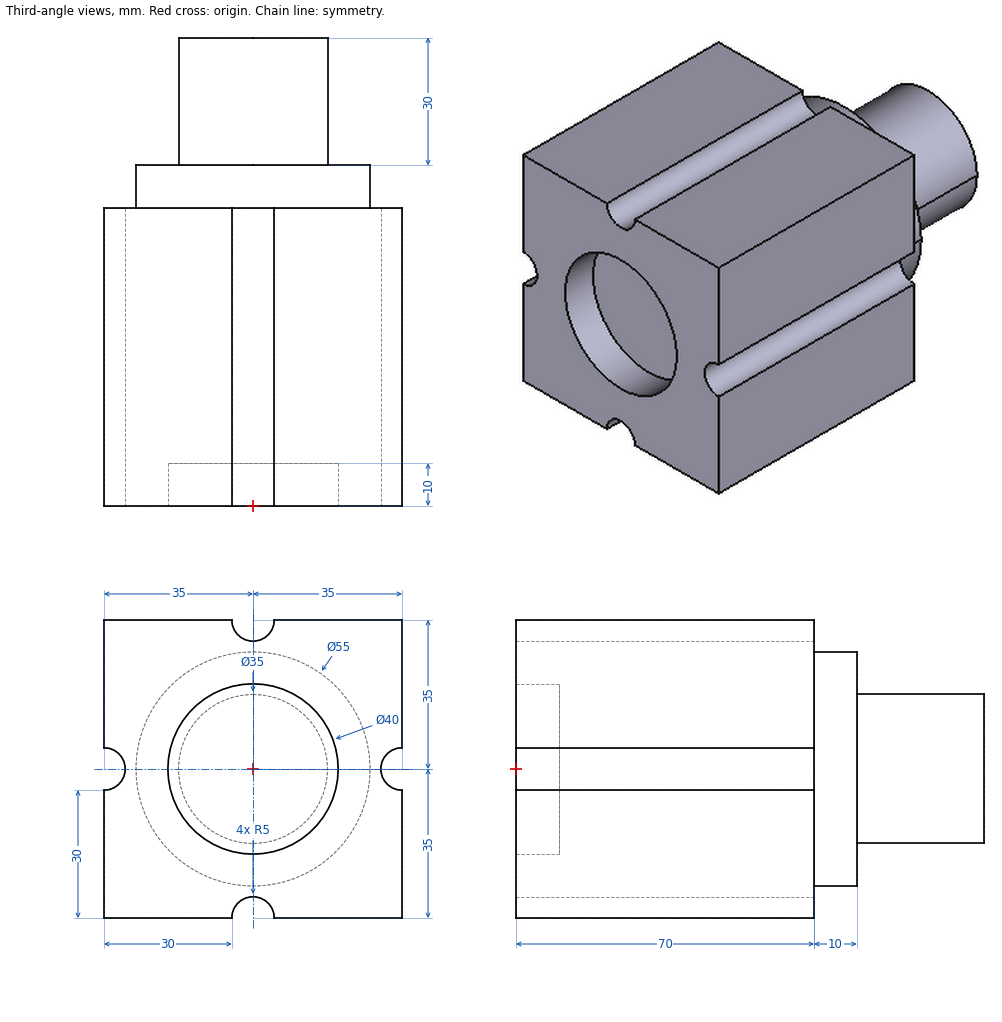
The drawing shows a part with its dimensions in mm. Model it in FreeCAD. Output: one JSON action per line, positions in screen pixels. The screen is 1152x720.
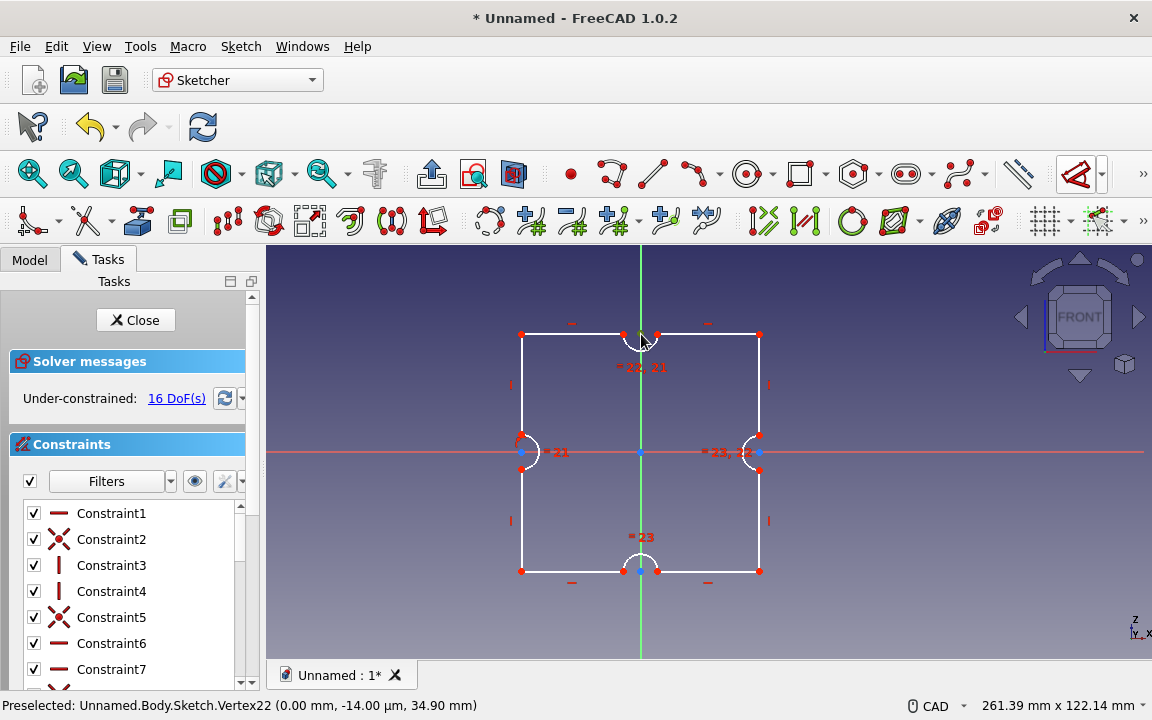
{"action": "left_click", "coordinate": [641, 605]}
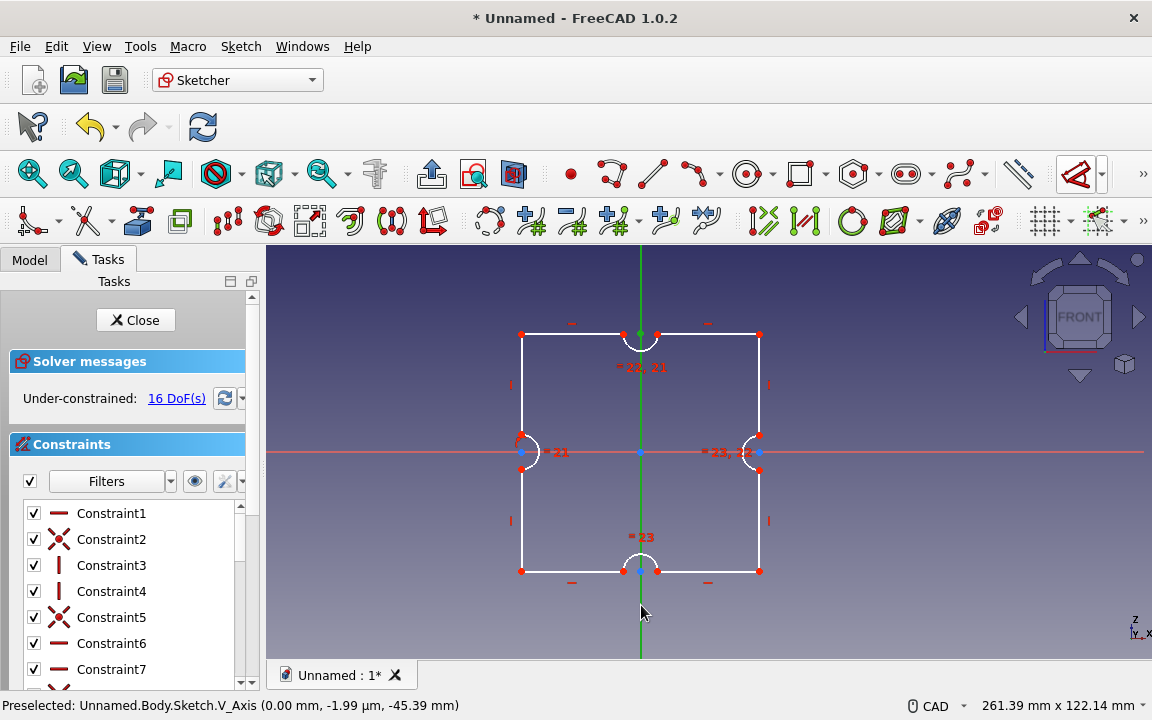
{"action": "key", "text": "c"}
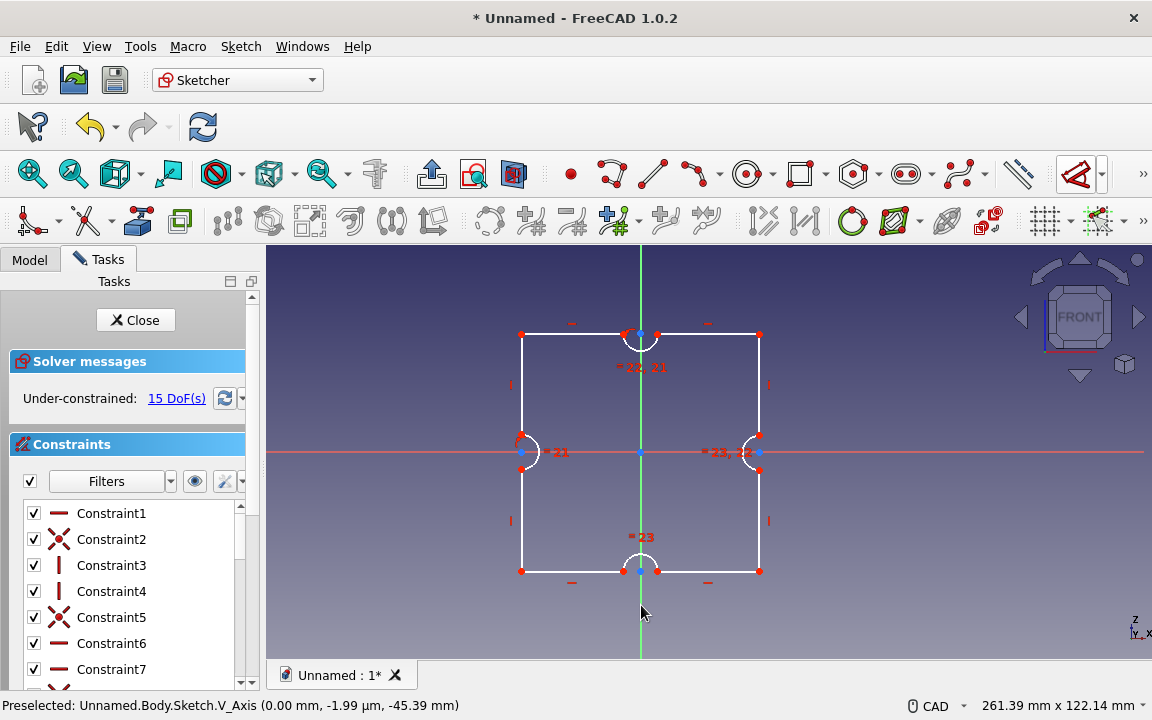
{"action": "left_click", "coordinate": [760, 453]}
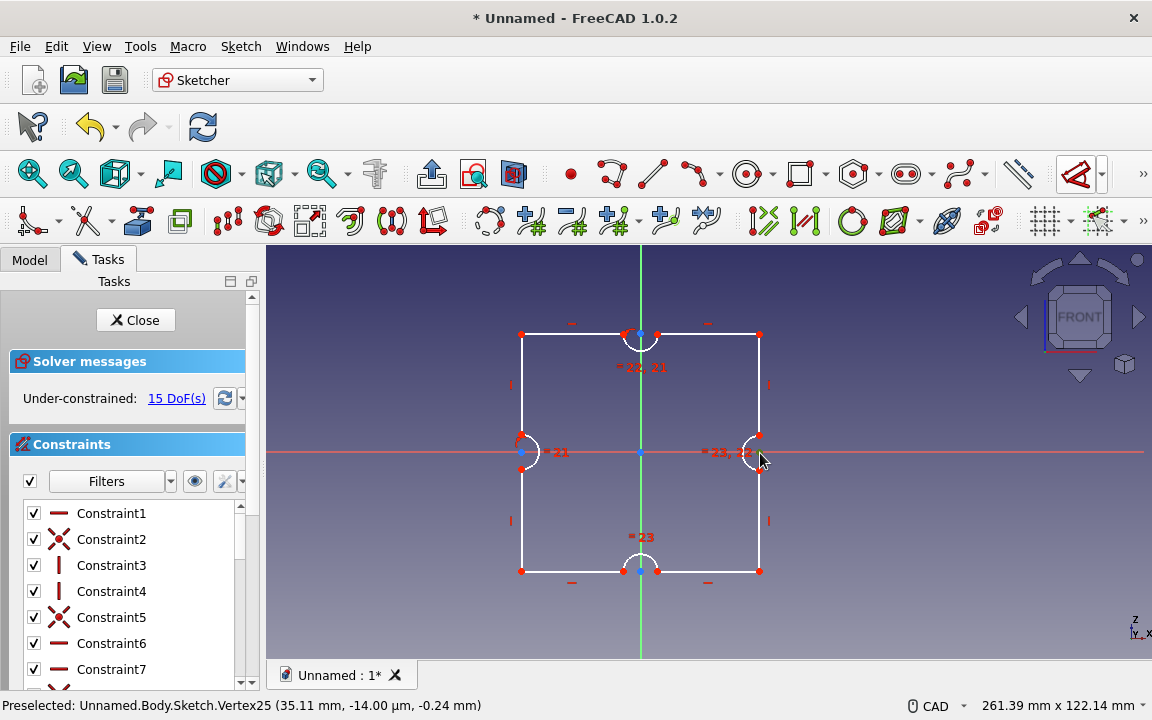
{"action": "left_click", "coordinate": [344, 452]}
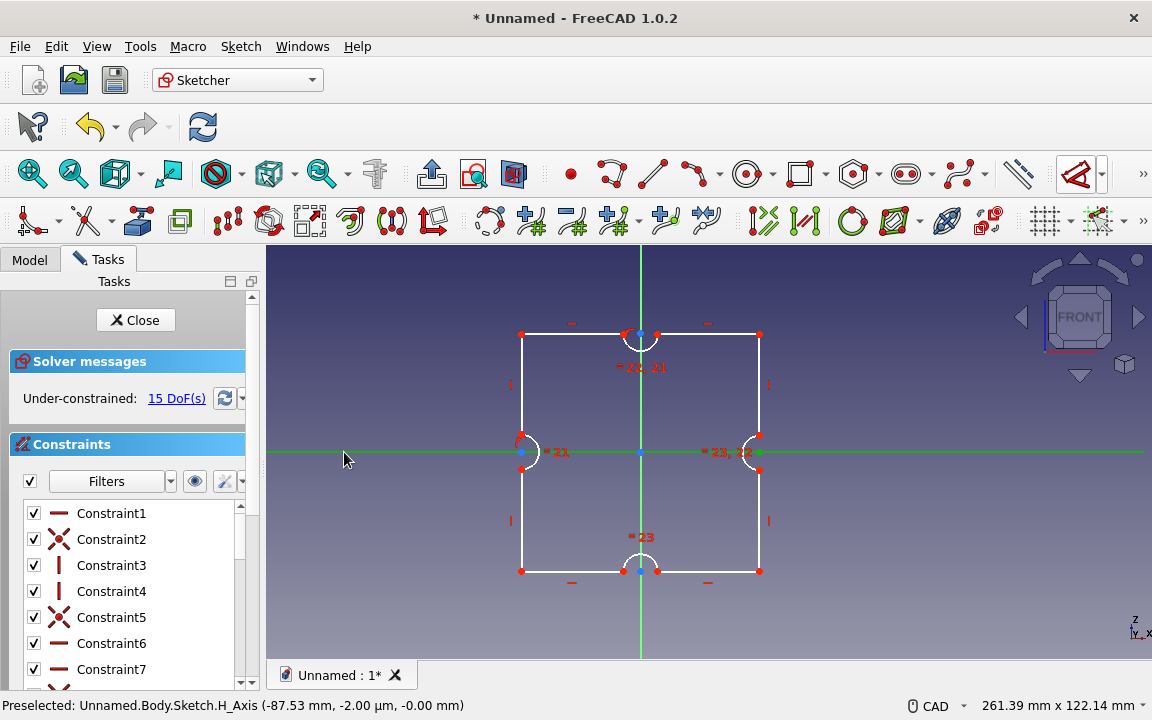
{"action": "key", "text": "c"}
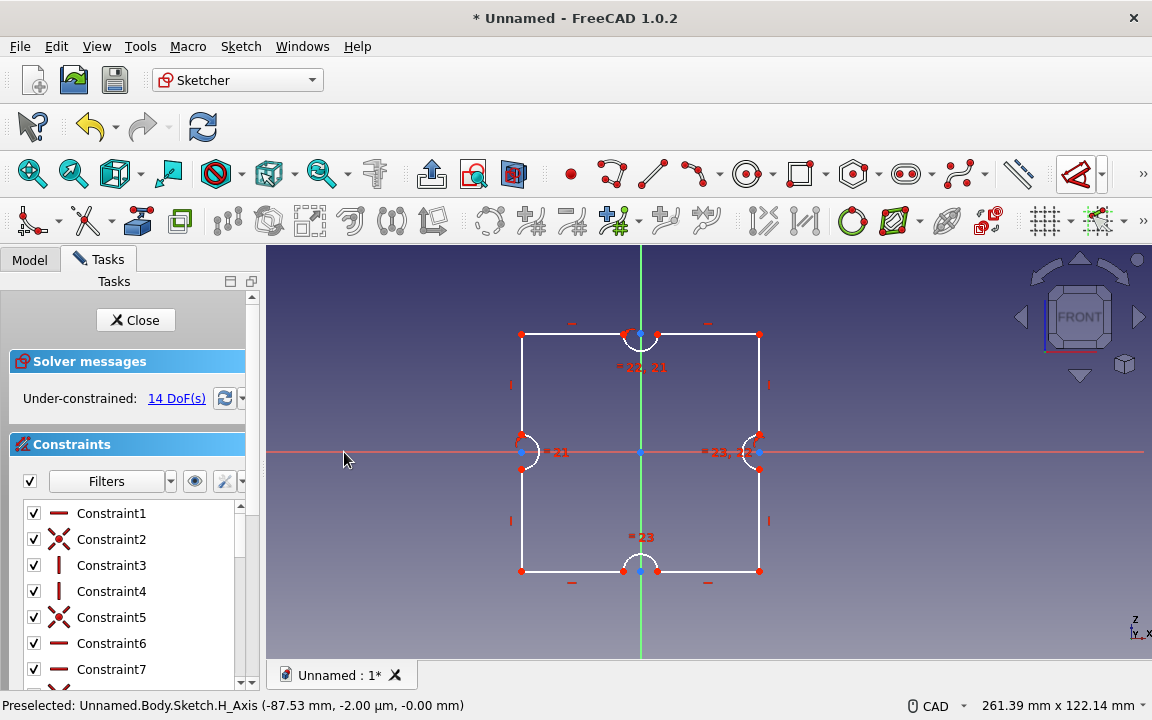
{"action": "left_click", "coordinate": [641, 571]}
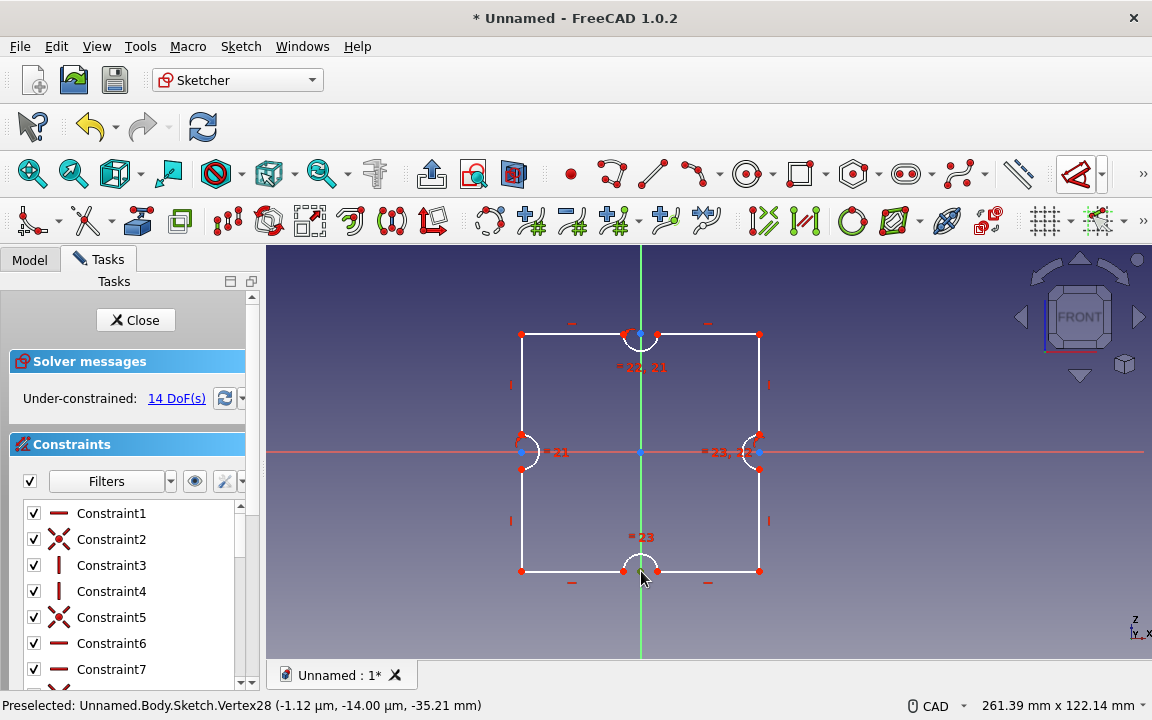
{"action": "left_click", "coordinate": [641, 605]}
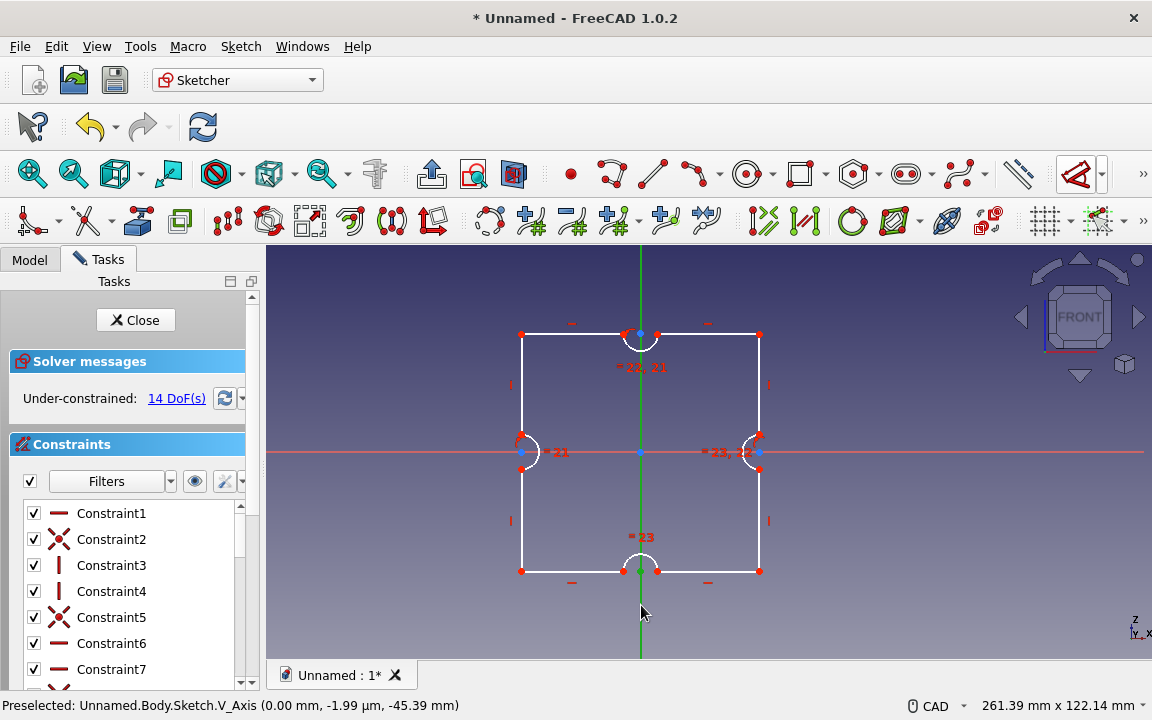
{"action": "key", "text": "c"}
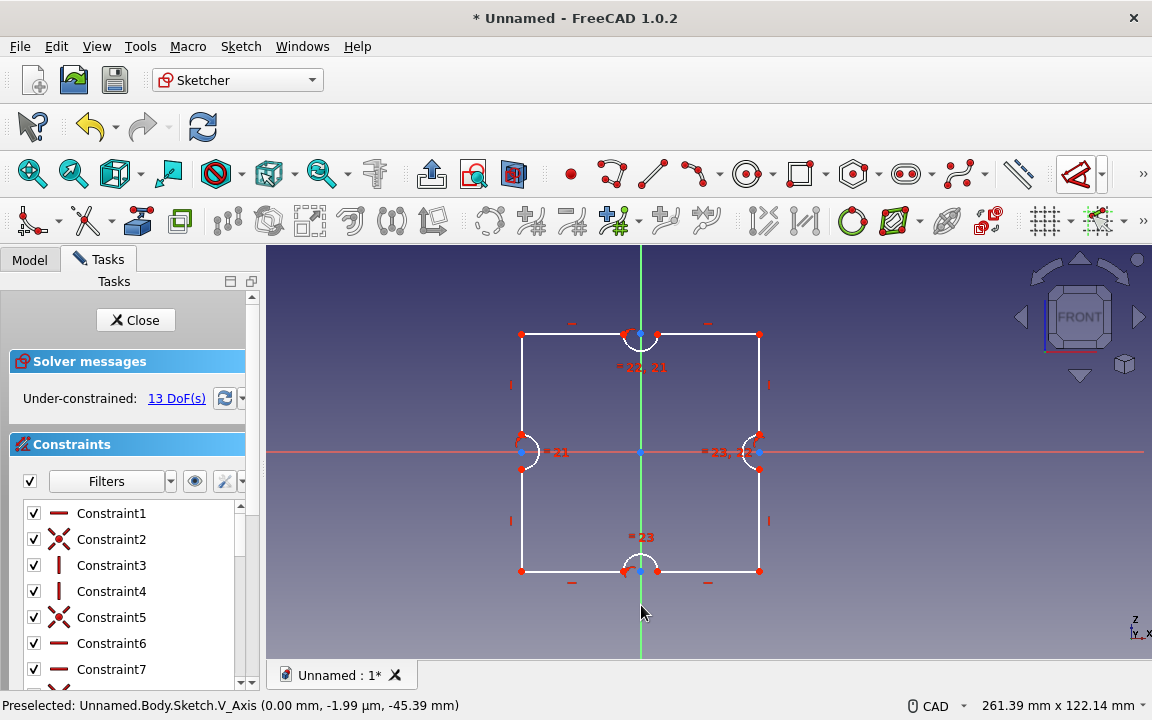
{"action": "left_click", "coordinate": [522, 572]}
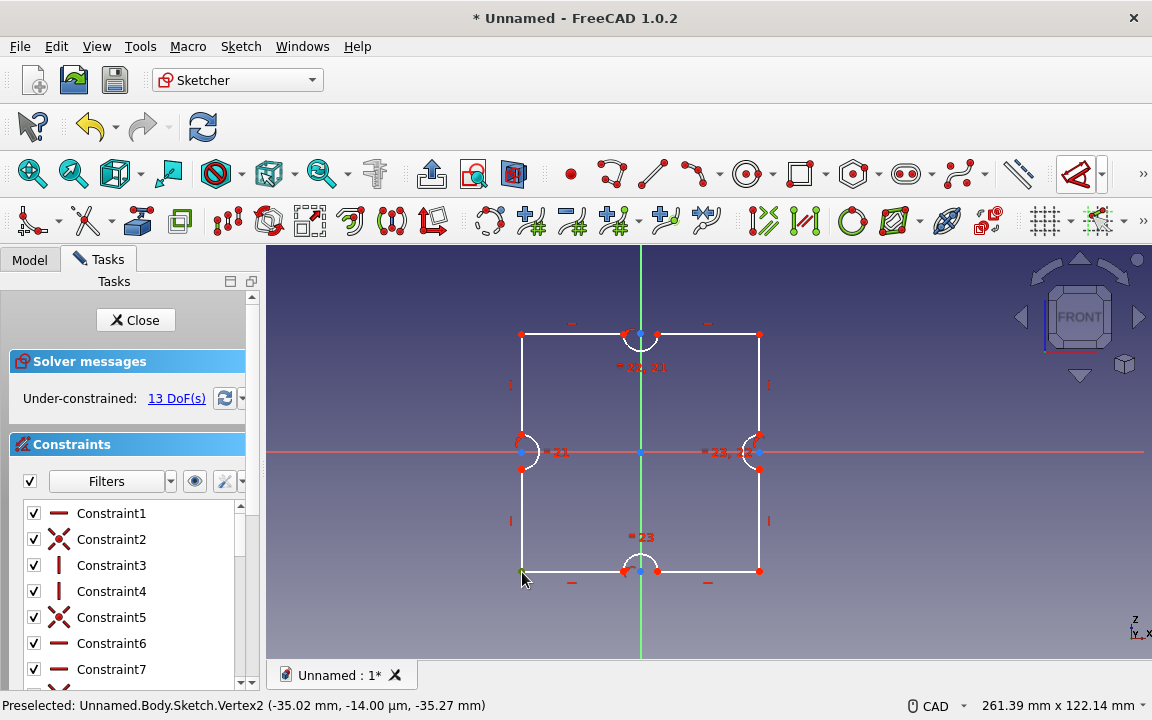
{"action": "left_click", "coordinate": [522, 334]}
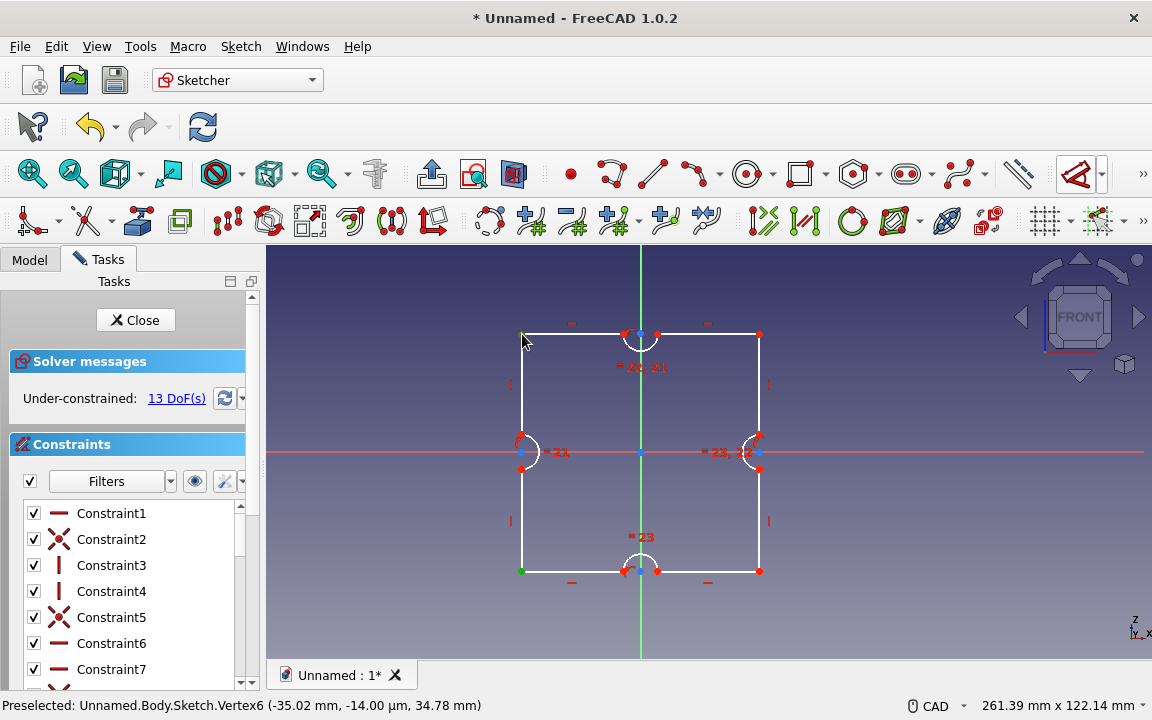
{"action": "left_click", "coordinate": [344, 452]}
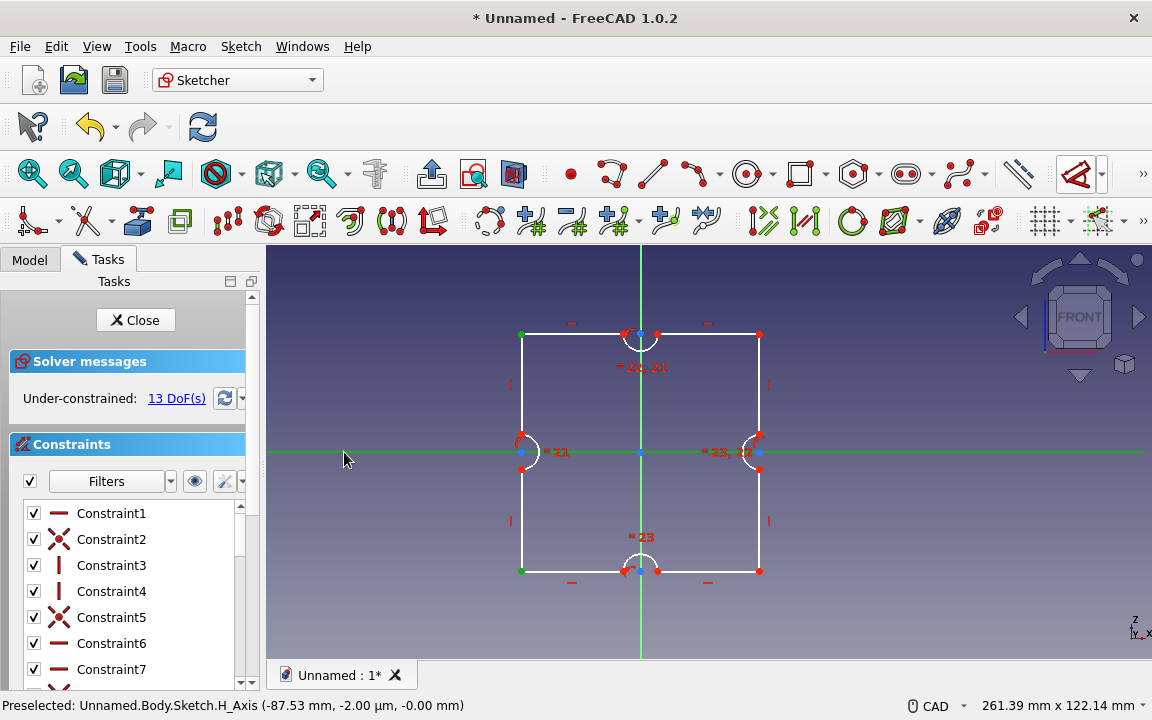
{"action": "key", "text": "s"}